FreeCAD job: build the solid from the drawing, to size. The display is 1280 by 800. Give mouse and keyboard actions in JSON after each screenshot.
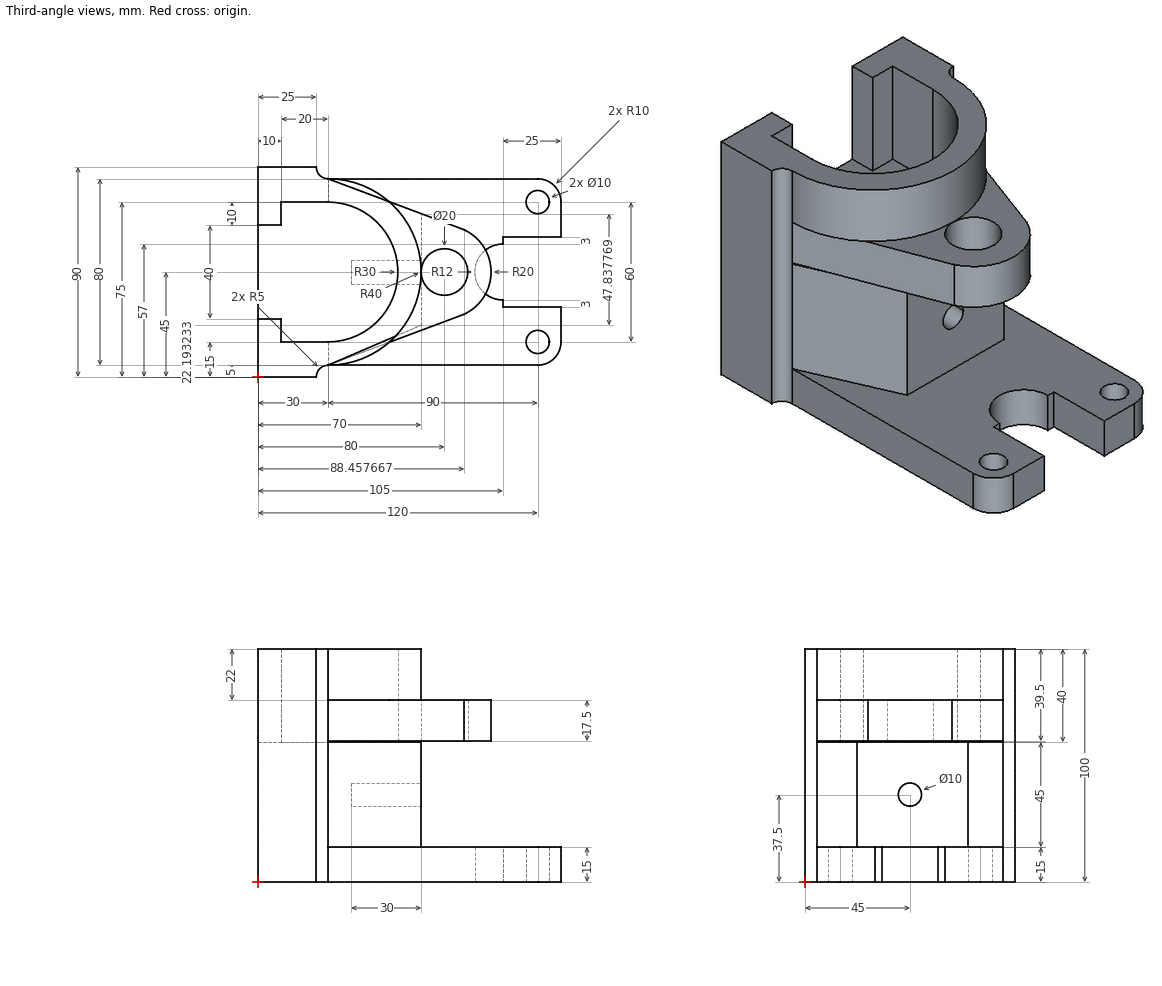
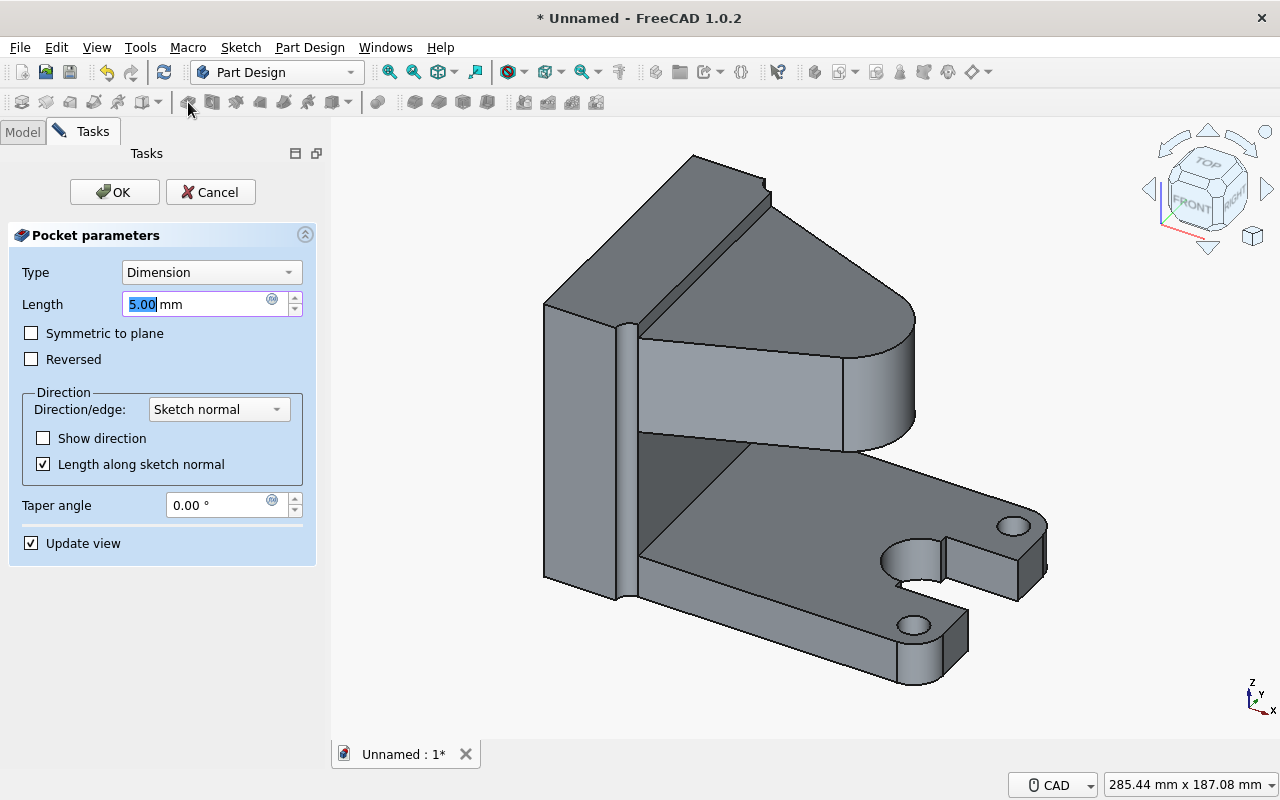
{"action": "type", "text": "22"}
{"action": "key", "text": "Tab"}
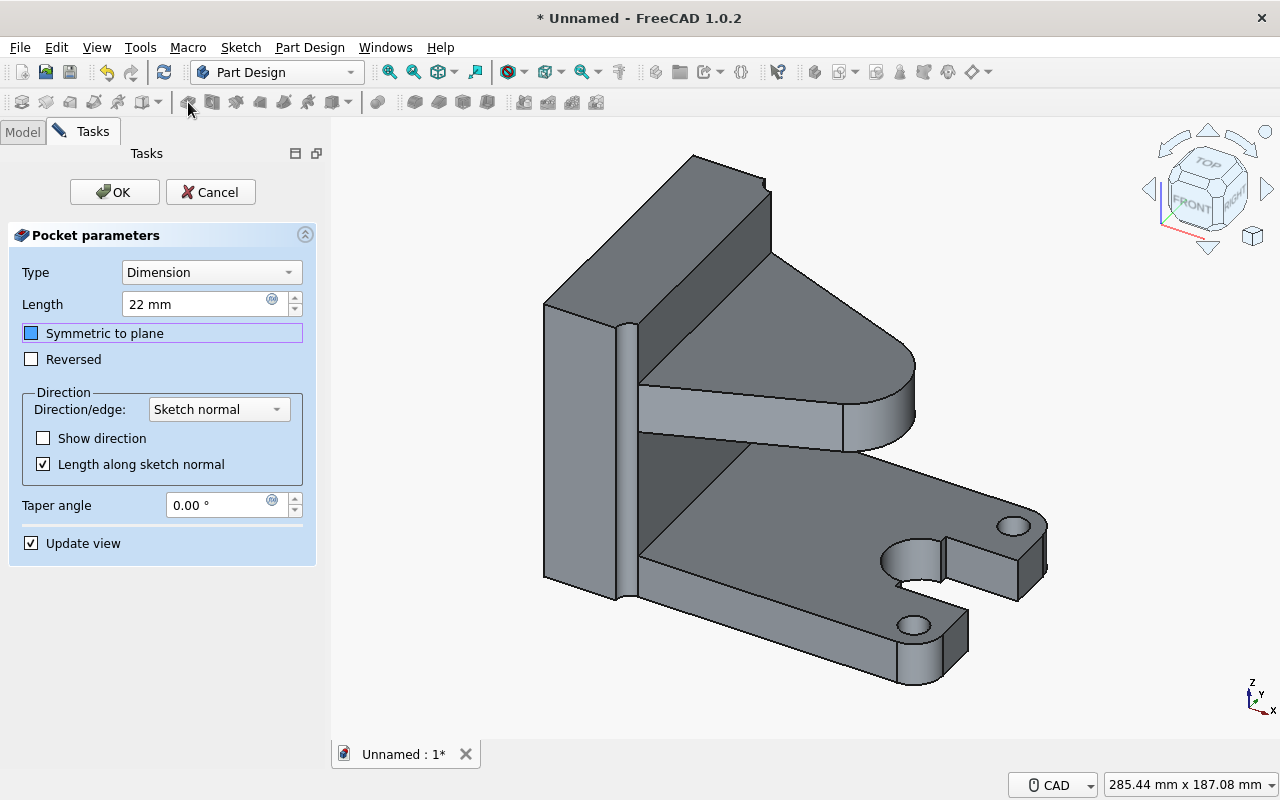
{"action": "left_click", "coordinate": [115, 192]}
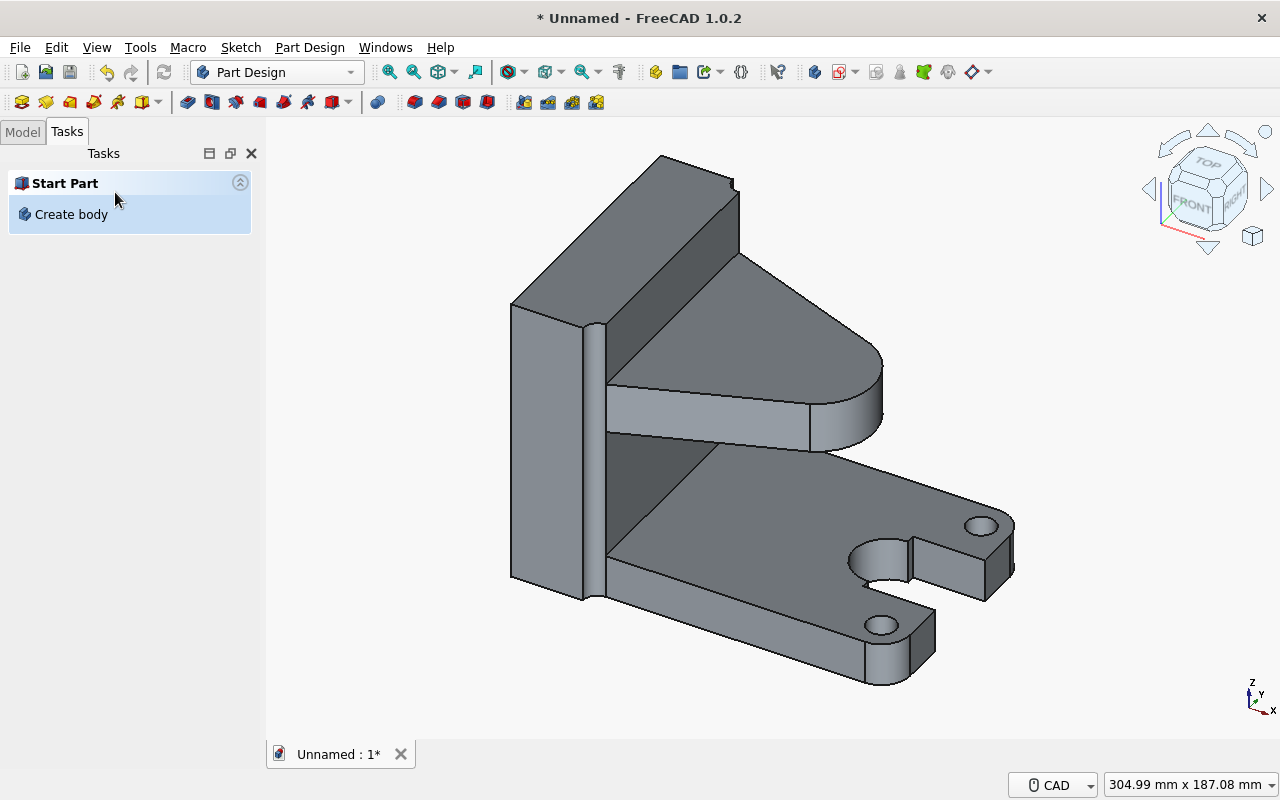
{"action": "left_click", "coordinate": [778, 574]}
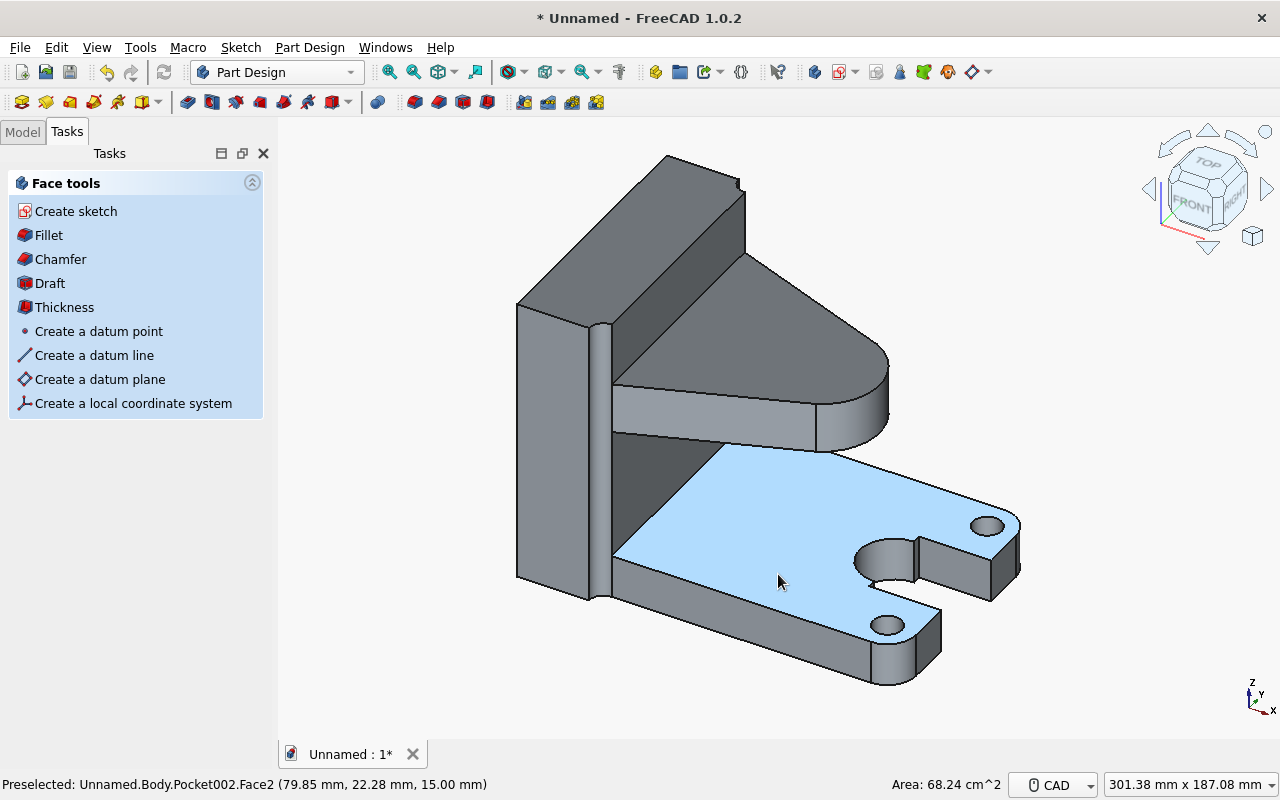
{"action": "left_click", "coordinate": [840, 72]}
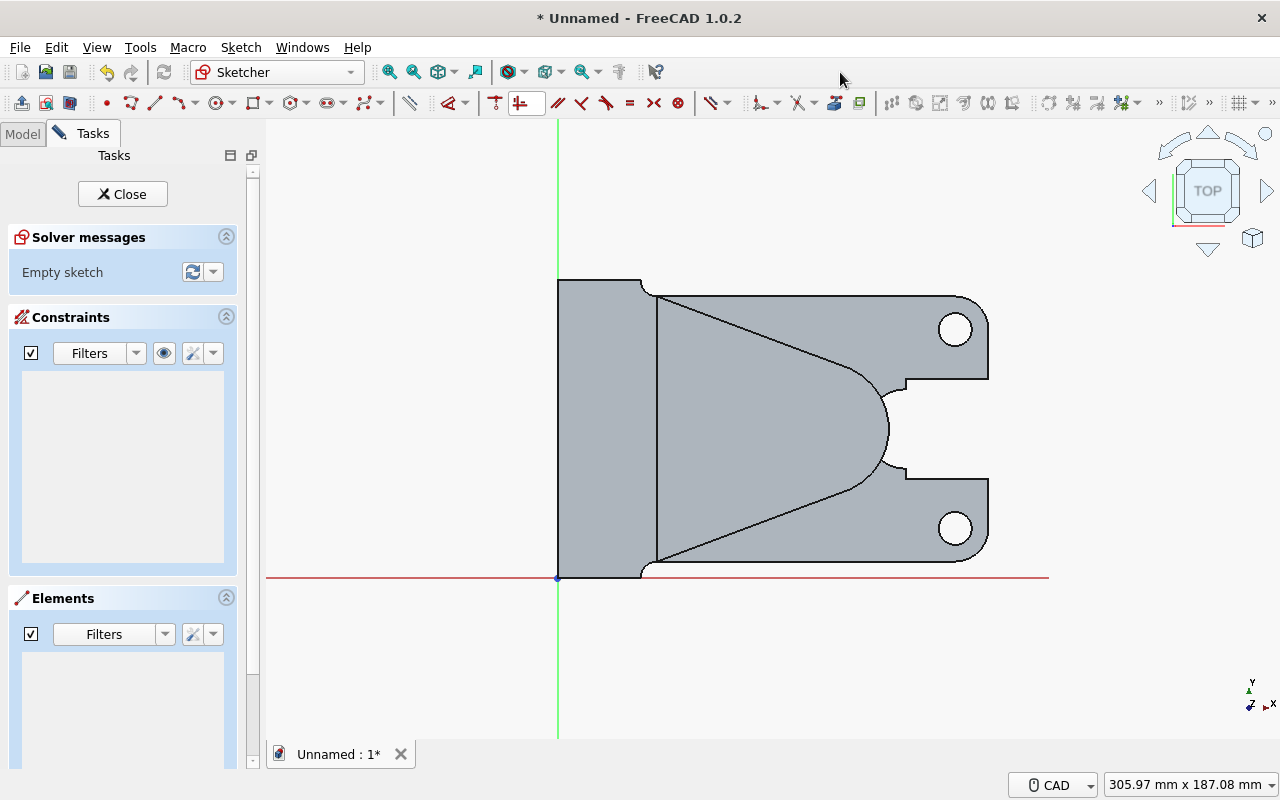
{"action": "scroll", "coordinate": [611, 454], "scroll_direction": "up", "scroll_amount": 2}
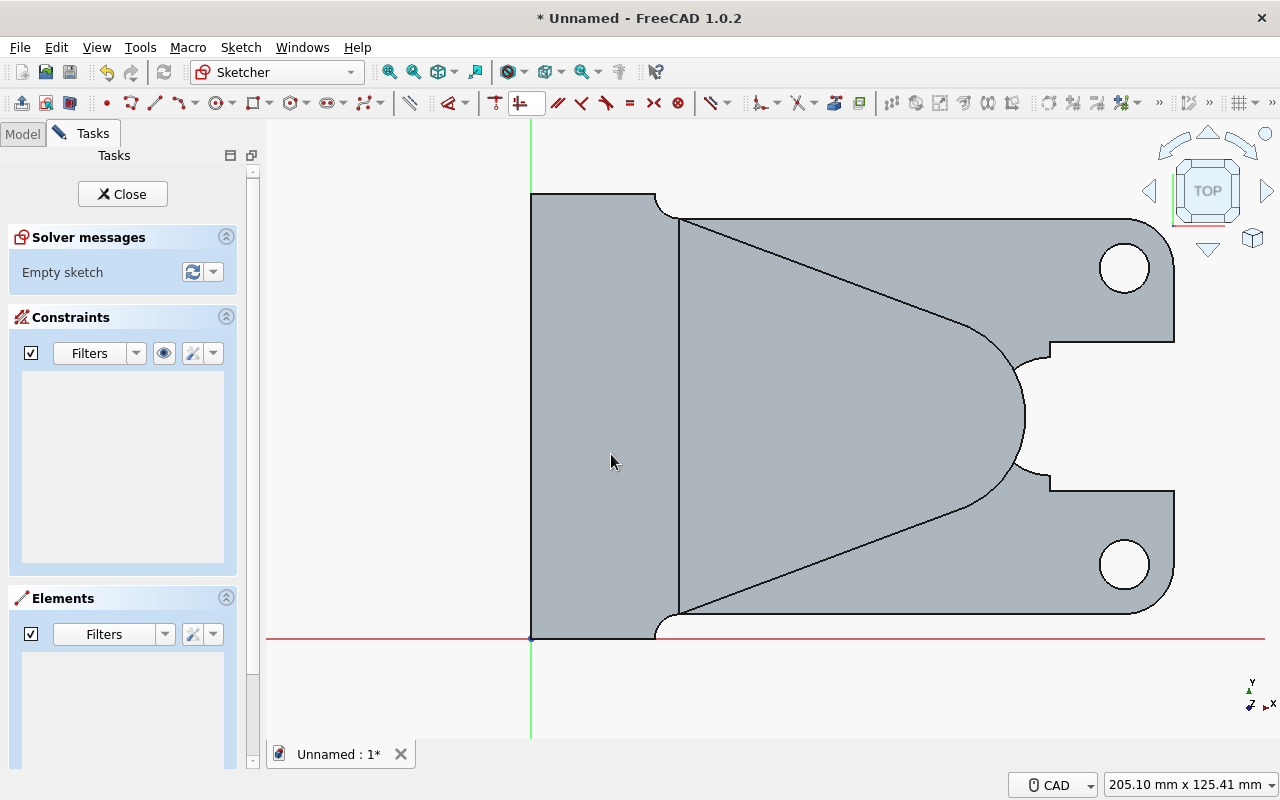
{"action": "key", "text": "g m"}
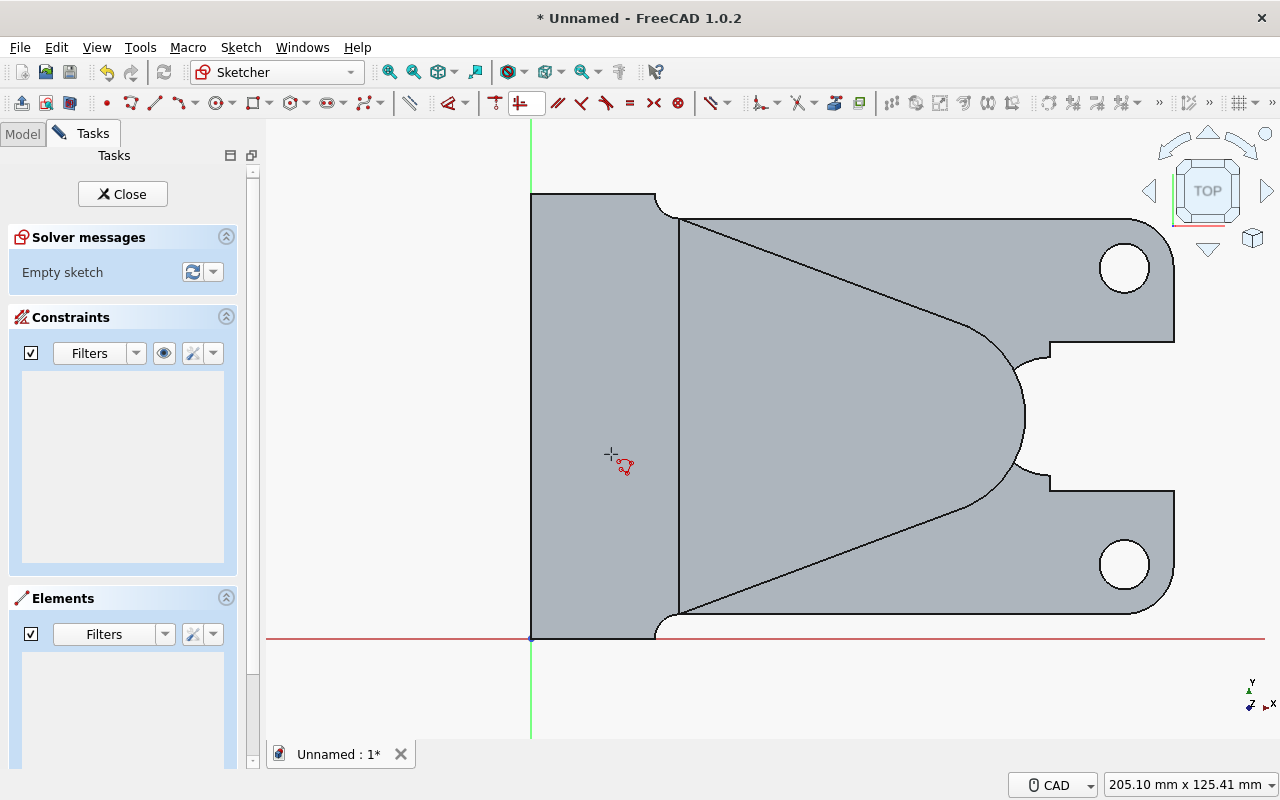
{"action": "left_click", "coordinate": [679, 614]}
{"action": "left_click", "coordinate": [877, 529]}
{"action": "left_click", "coordinate": [877, 293]}
{"action": "left_click", "coordinate": [679, 219]}
{"action": "left_click", "coordinate": [679, 615]}
{"action": "key", "text": "Escape"}
{"action": "key", "text": "Escape"}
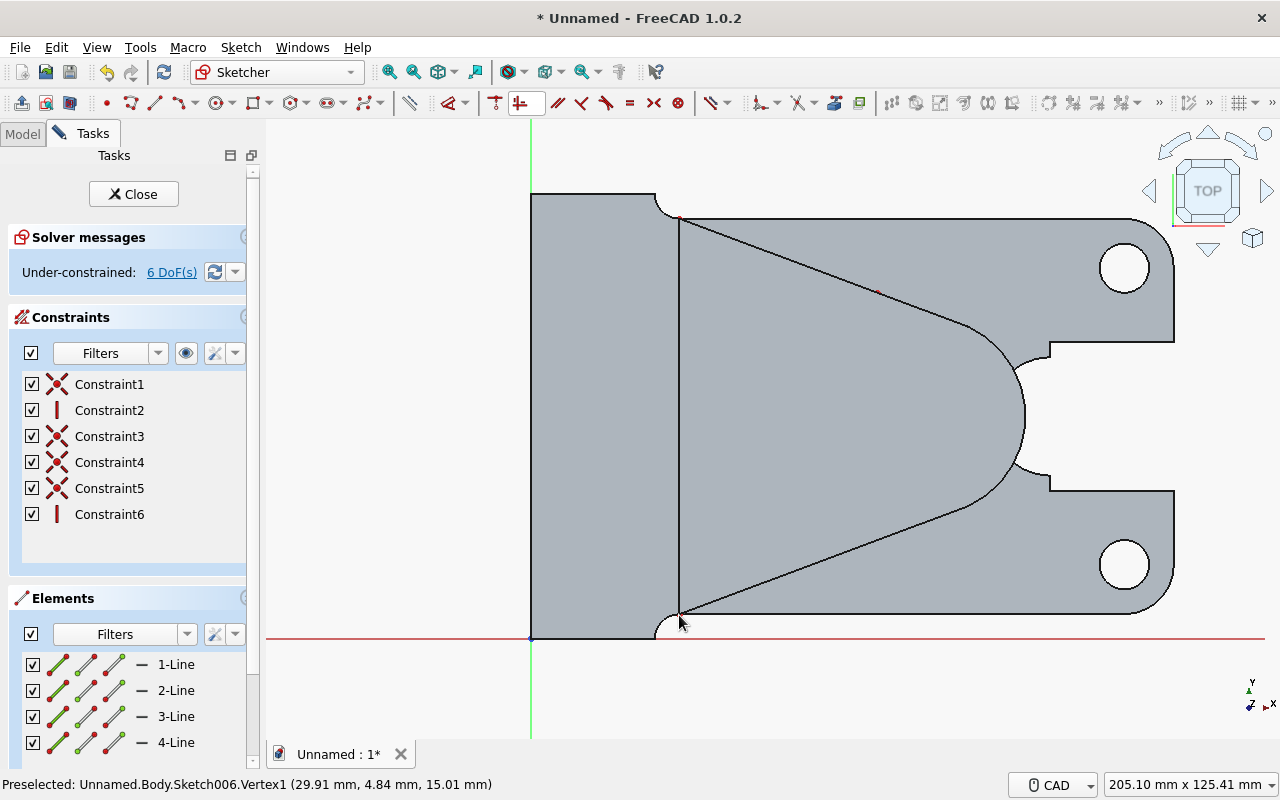
{"action": "key", "text": "d"}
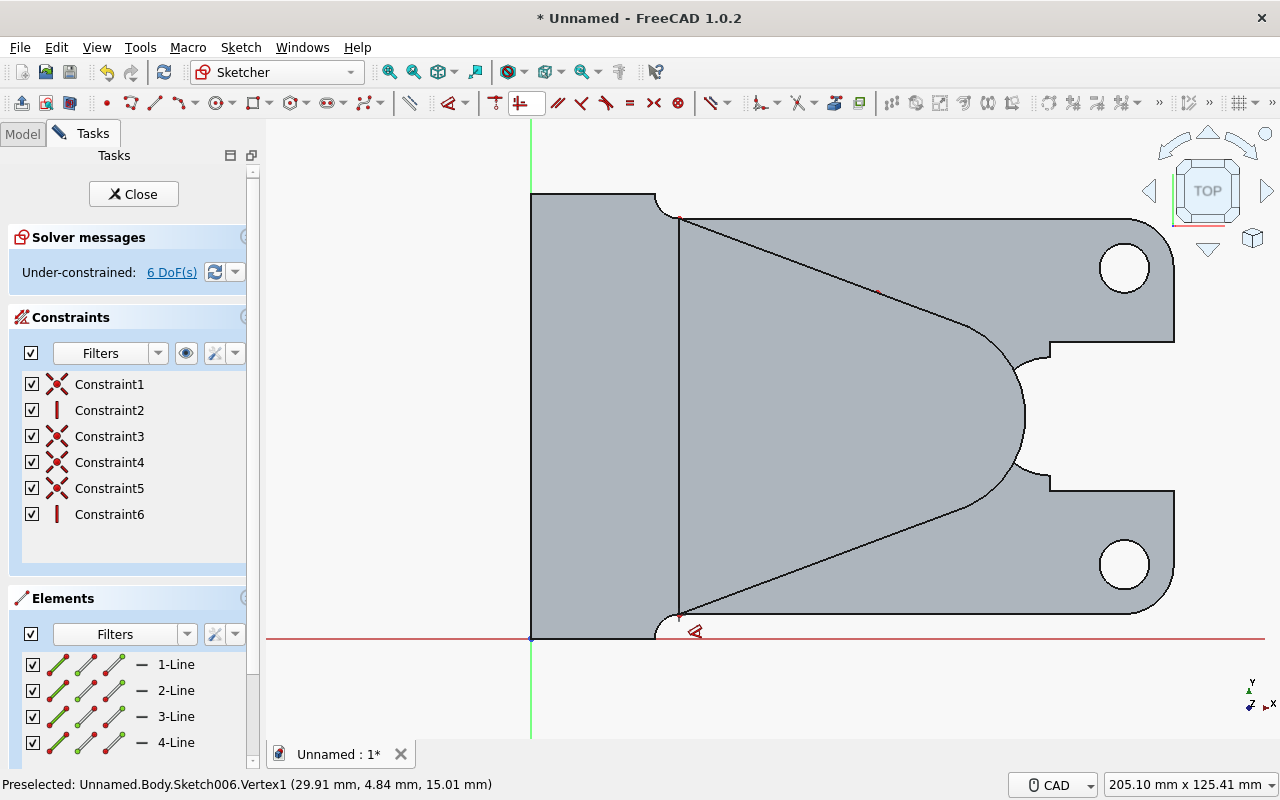
{"action": "left_click", "coordinate": [679, 339]}
{"action": "left_click", "coordinate": [645, 418]}